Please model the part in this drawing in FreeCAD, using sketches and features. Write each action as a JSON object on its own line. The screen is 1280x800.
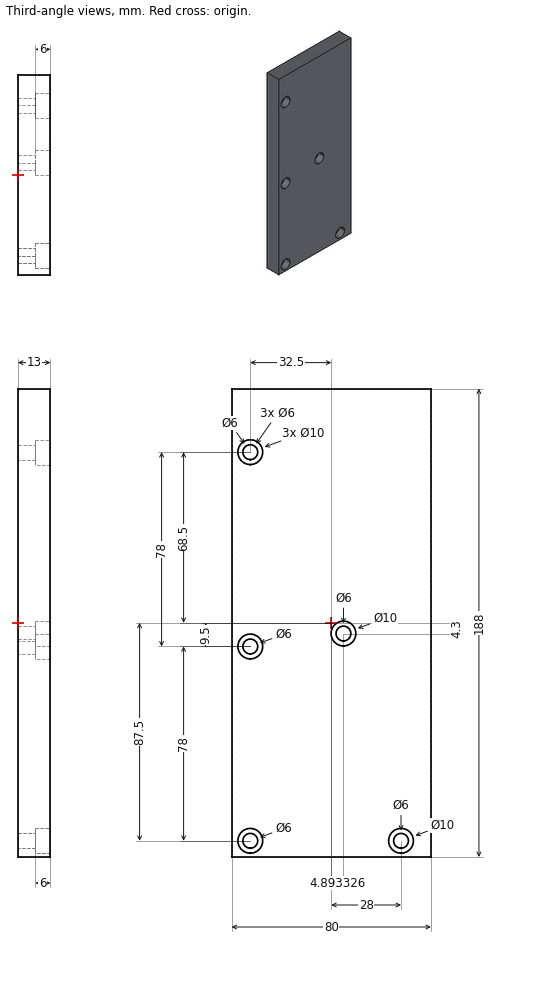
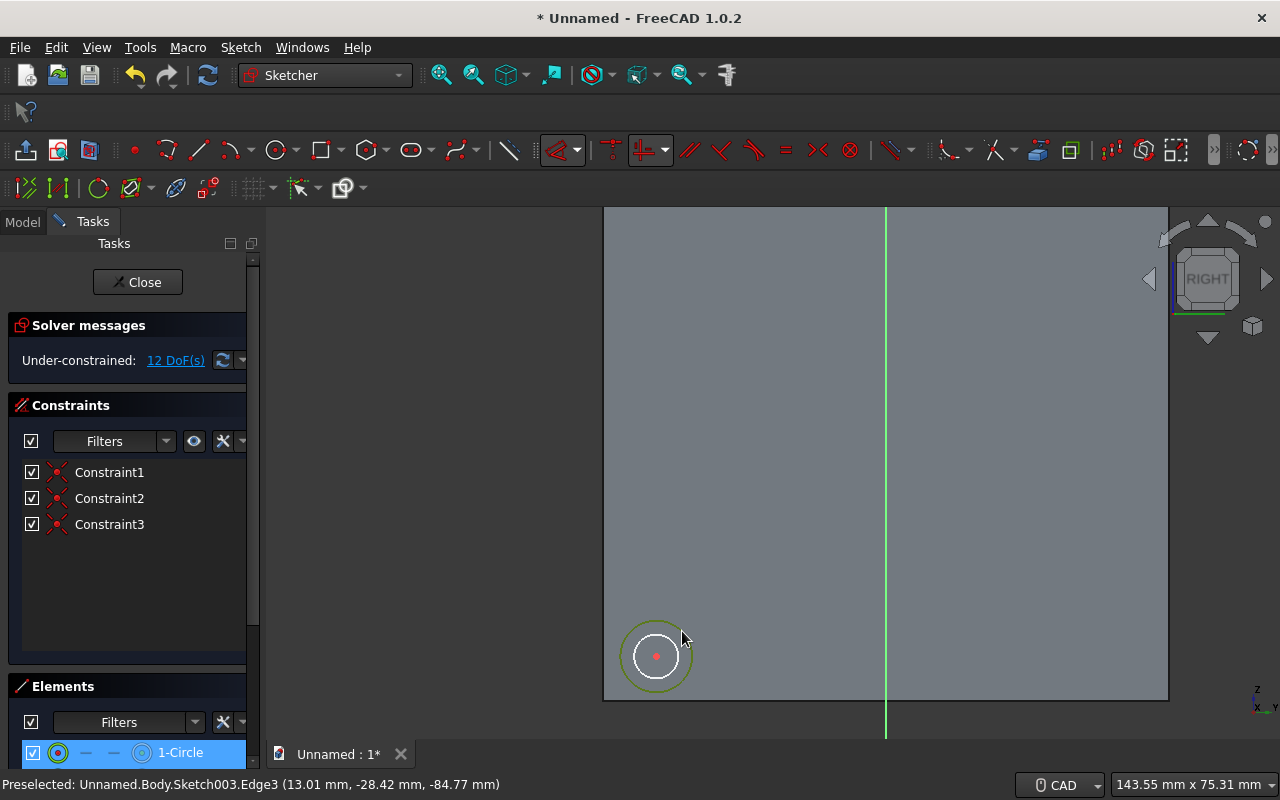
{"action": "left_click", "coordinate": [786, 150]}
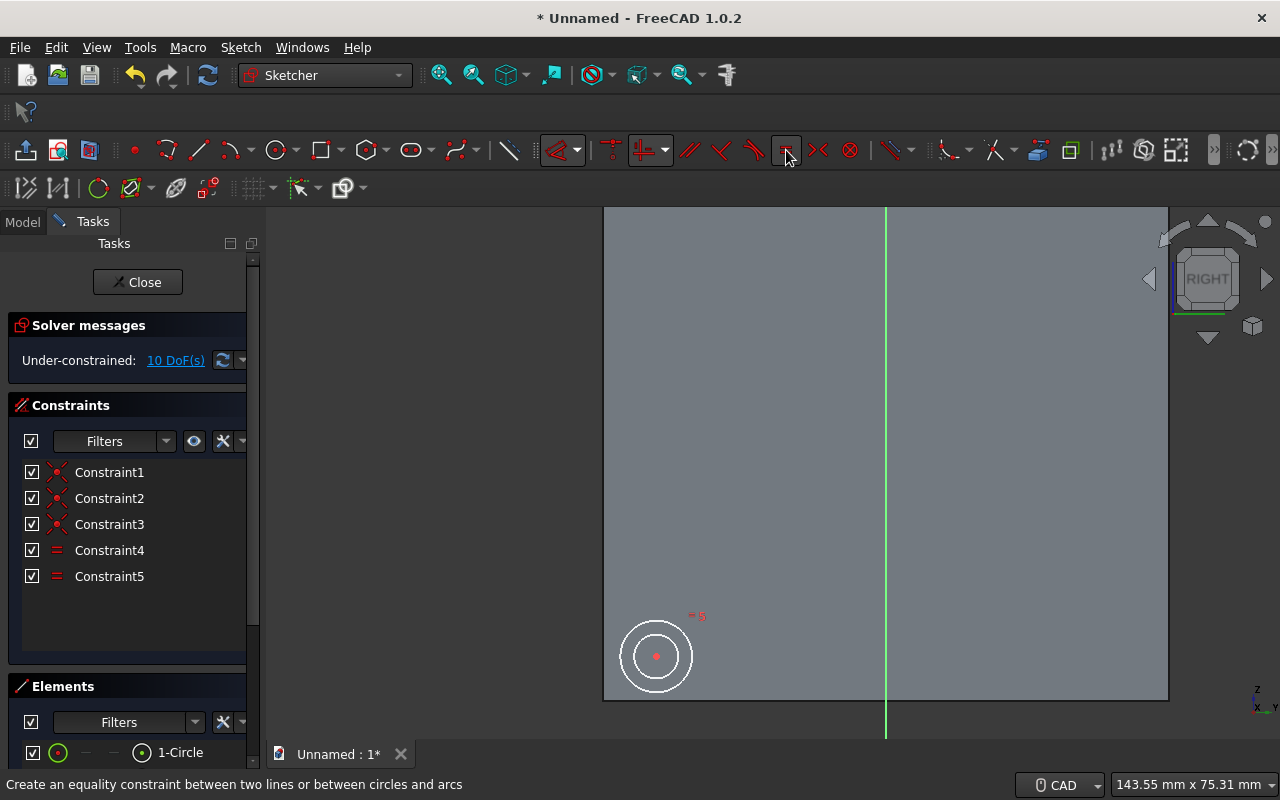
{"action": "scroll", "coordinate": [683, 632], "scroll_direction": "down", "scroll_amount": 6}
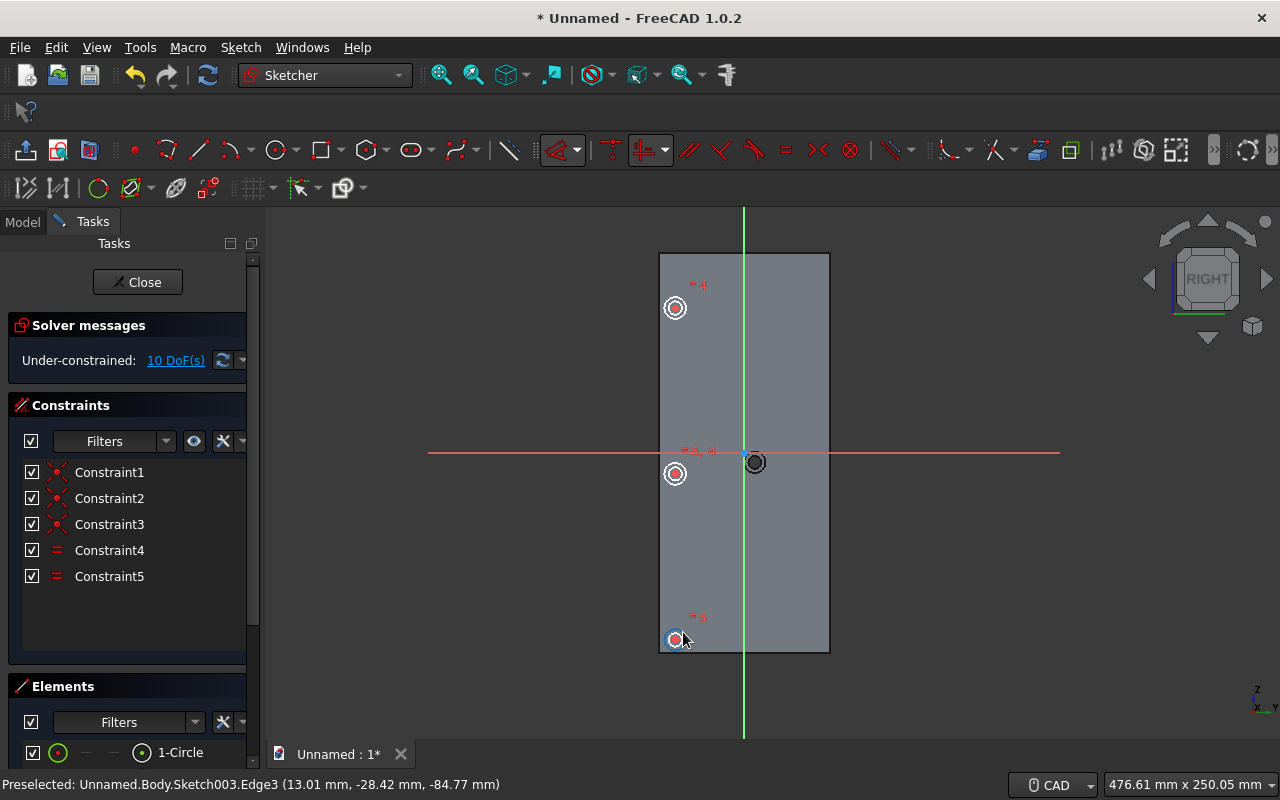
{"action": "scroll", "coordinate": [680, 303], "scroll_direction": "up", "scroll_amount": 7}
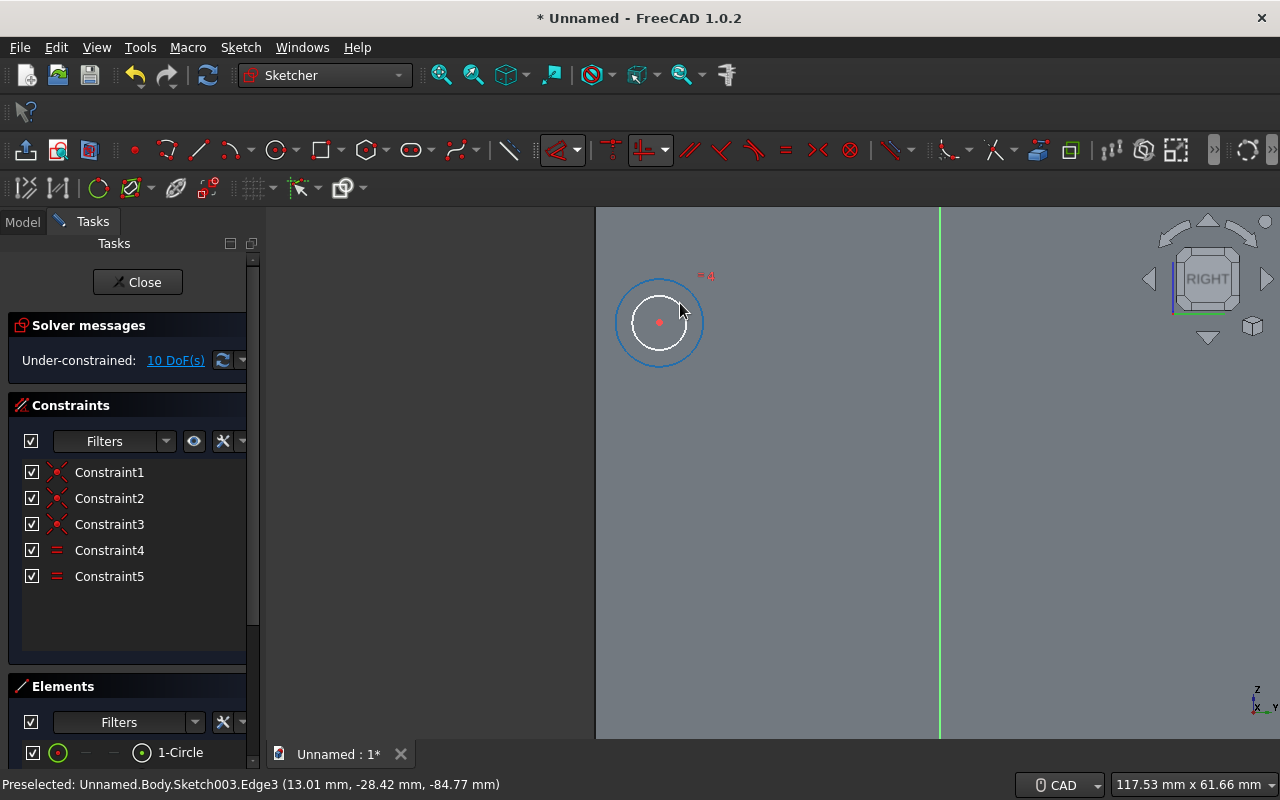
{"action": "left_click", "coordinate": [678, 304]}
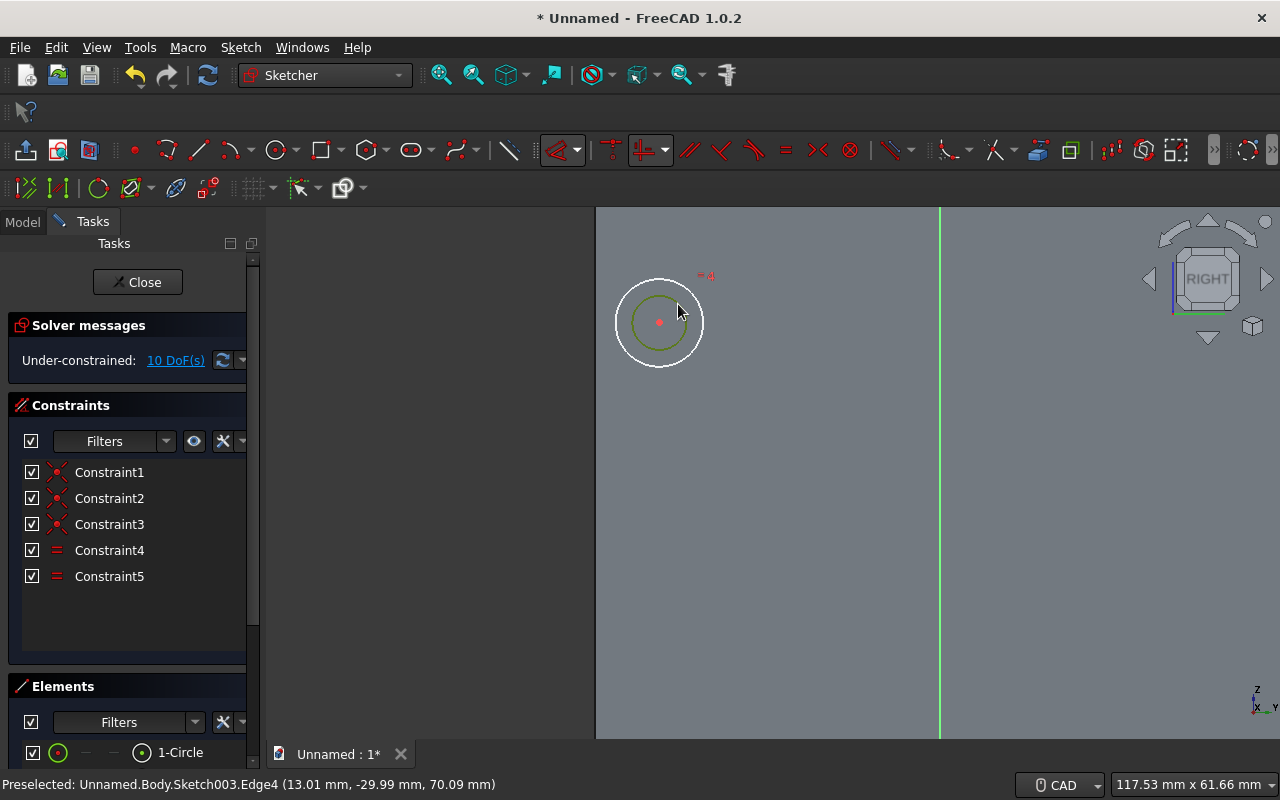
{"action": "scroll", "coordinate": [680, 303], "scroll_direction": "down", "scroll_amount": 7}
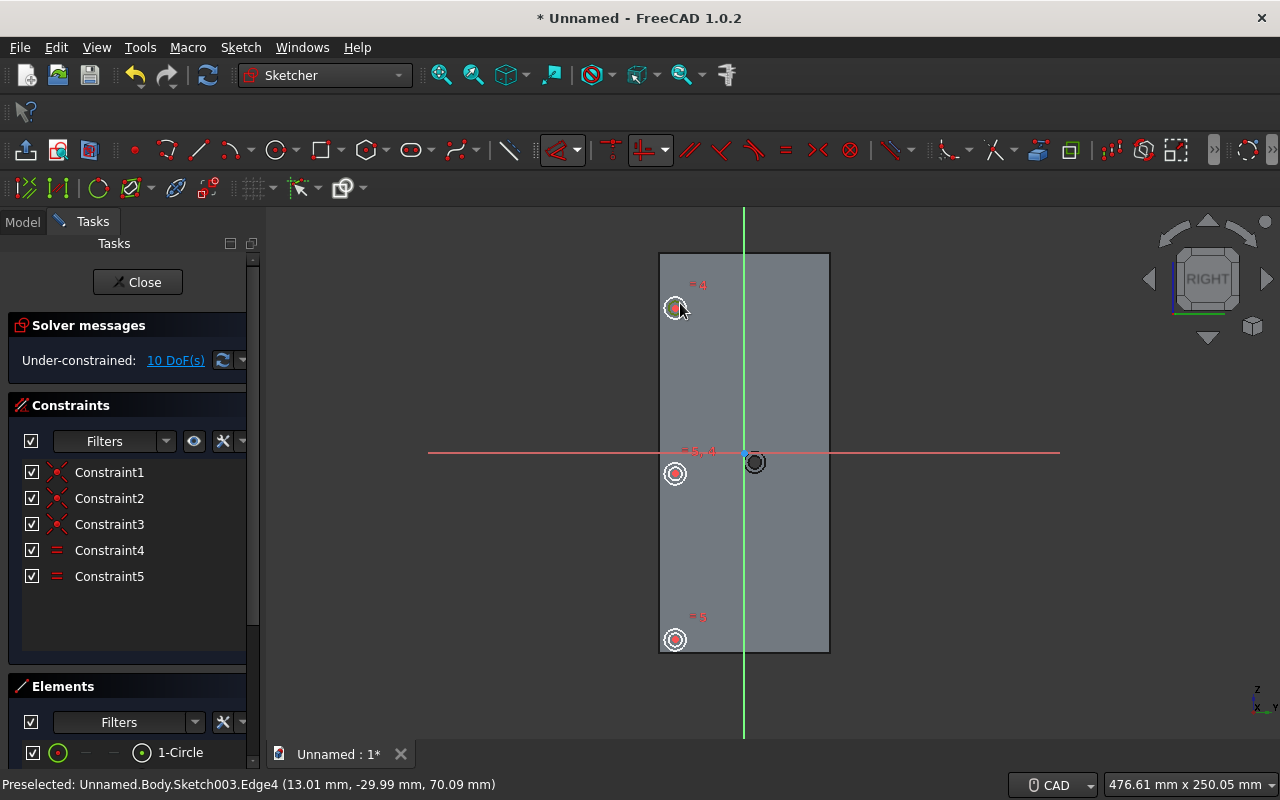
{"action": "scroll", "coordinate": [680, 469], "scroll_direction": "up", "scroll_amount": 6}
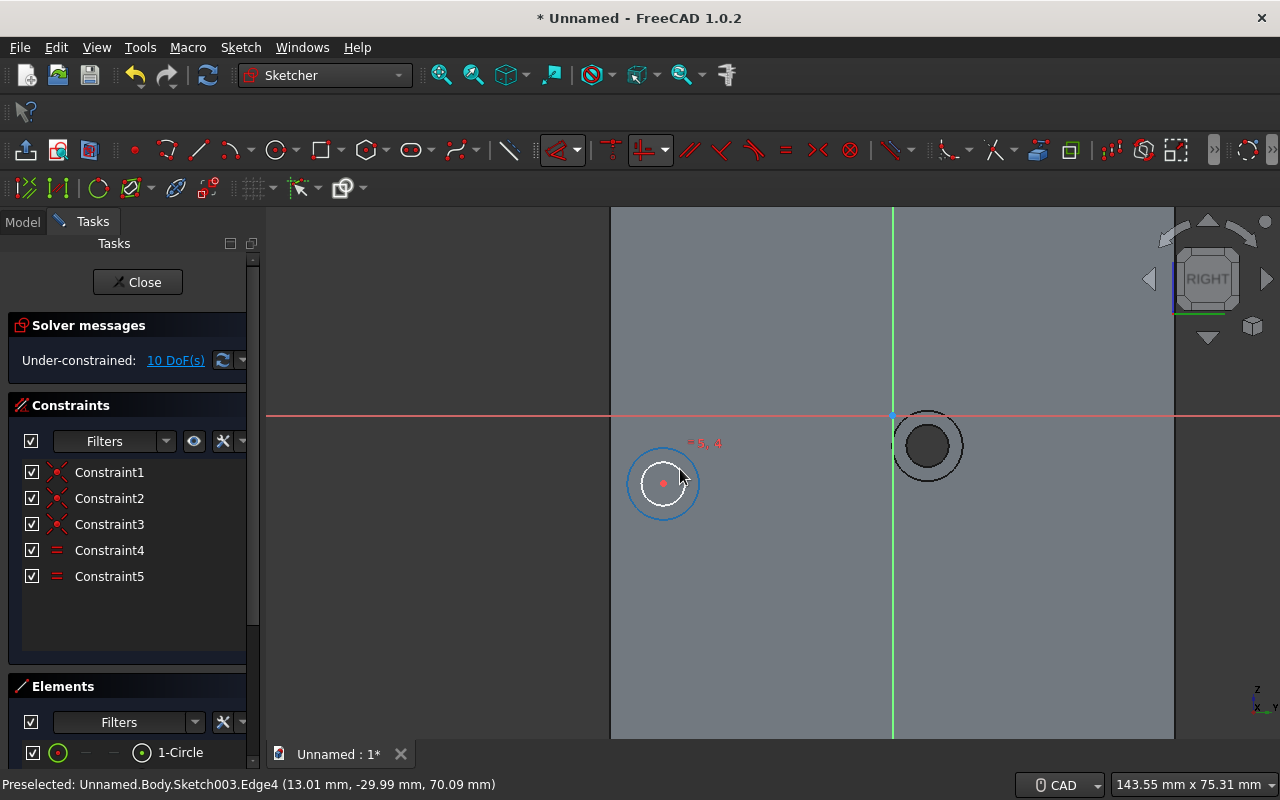
{"action": "left_click", "coordinate": [678, 469]}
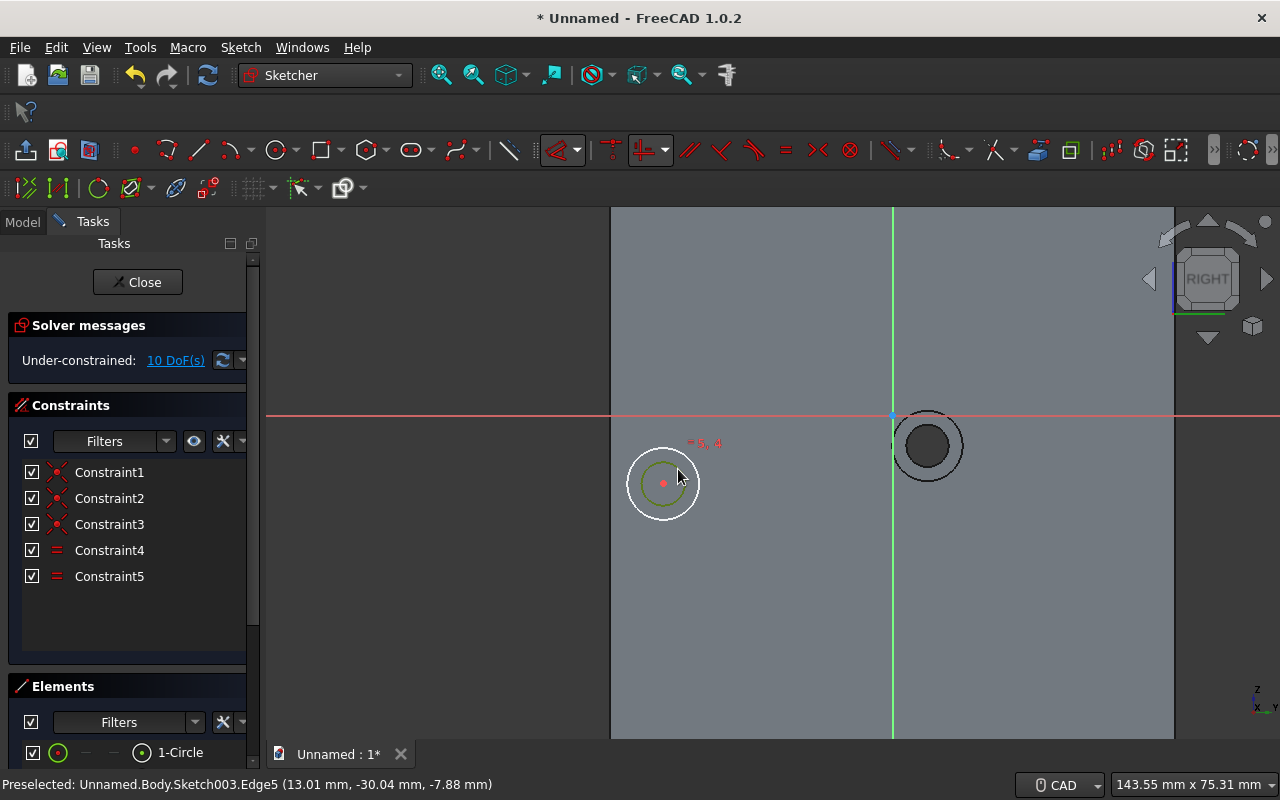
{"action": "scroll", "coordinate": [680, 469], "scroll_direction": "down", "scroll_amount": 6}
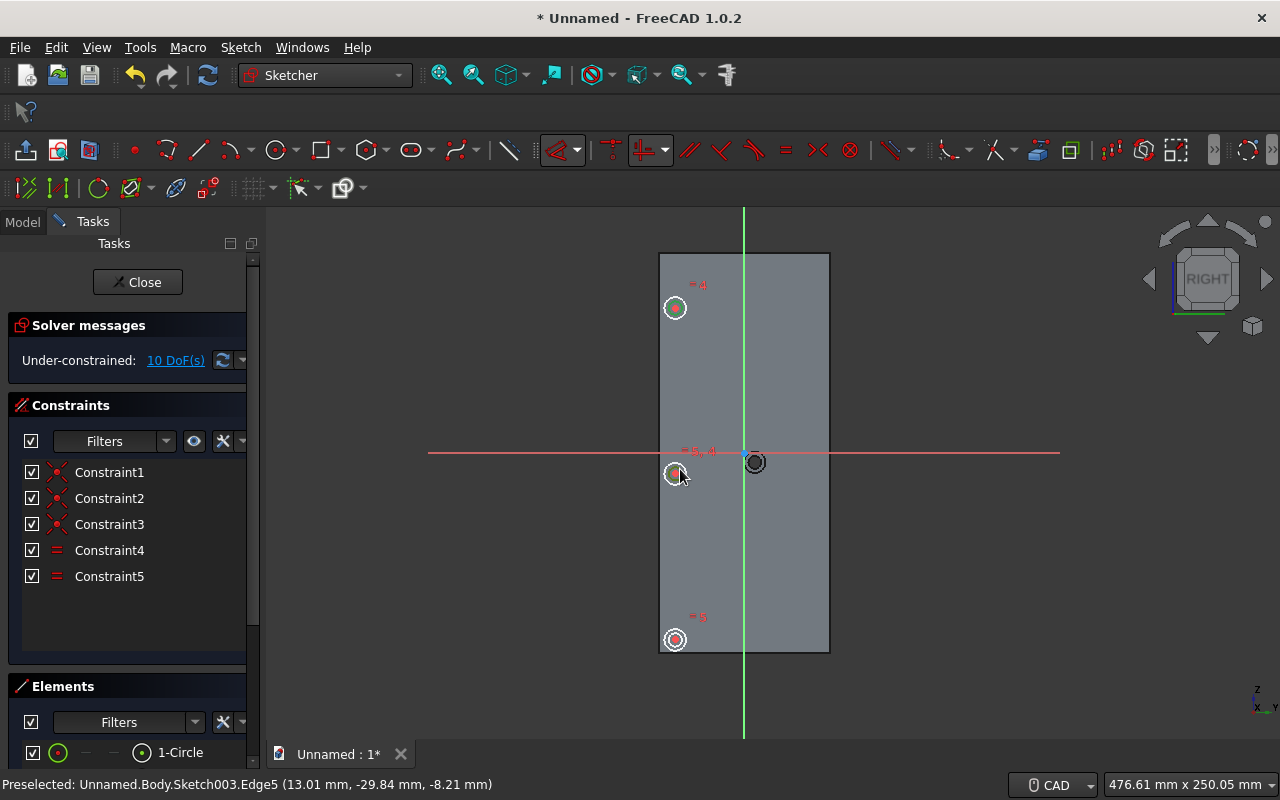
{"action": "scroll", "coordinate": [680, 635], "scroll_direction": "up", "scroll_amount": 6}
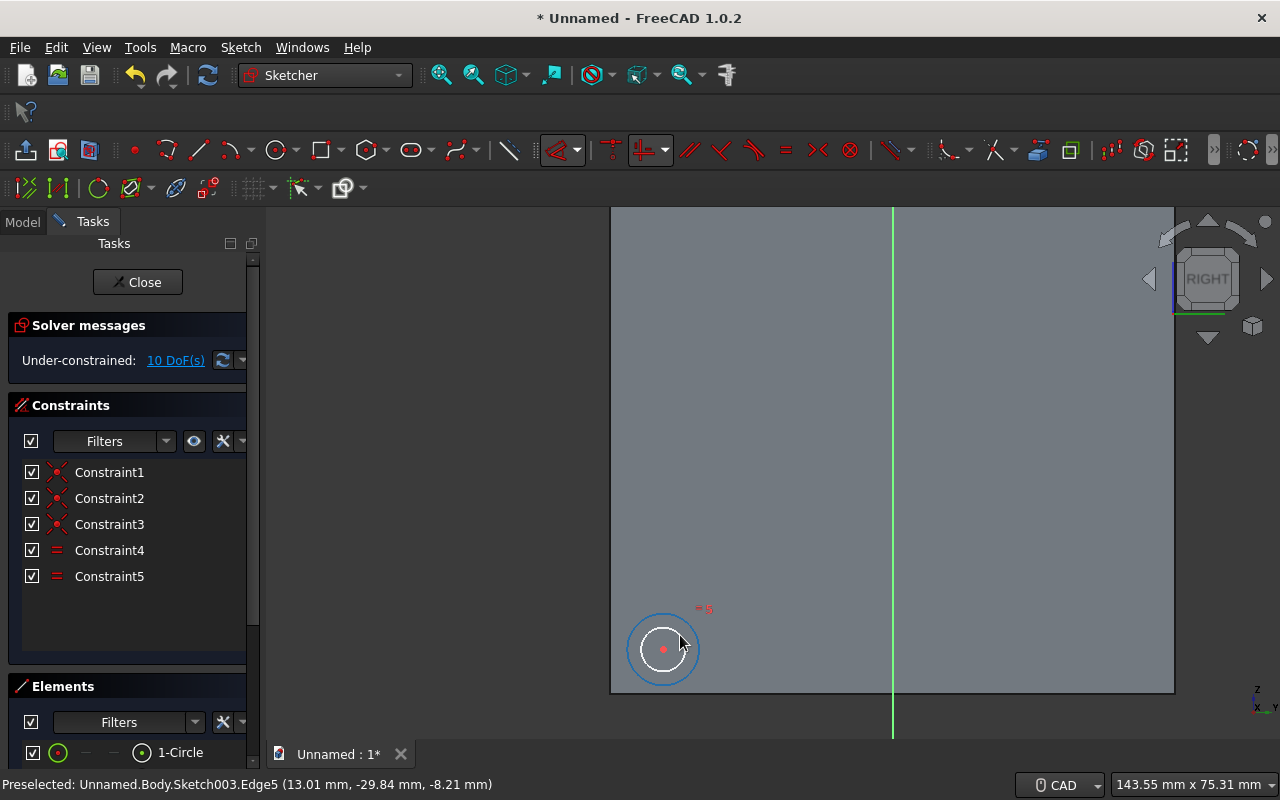
{"action": "left_click", "coordinate": [679, 634]}